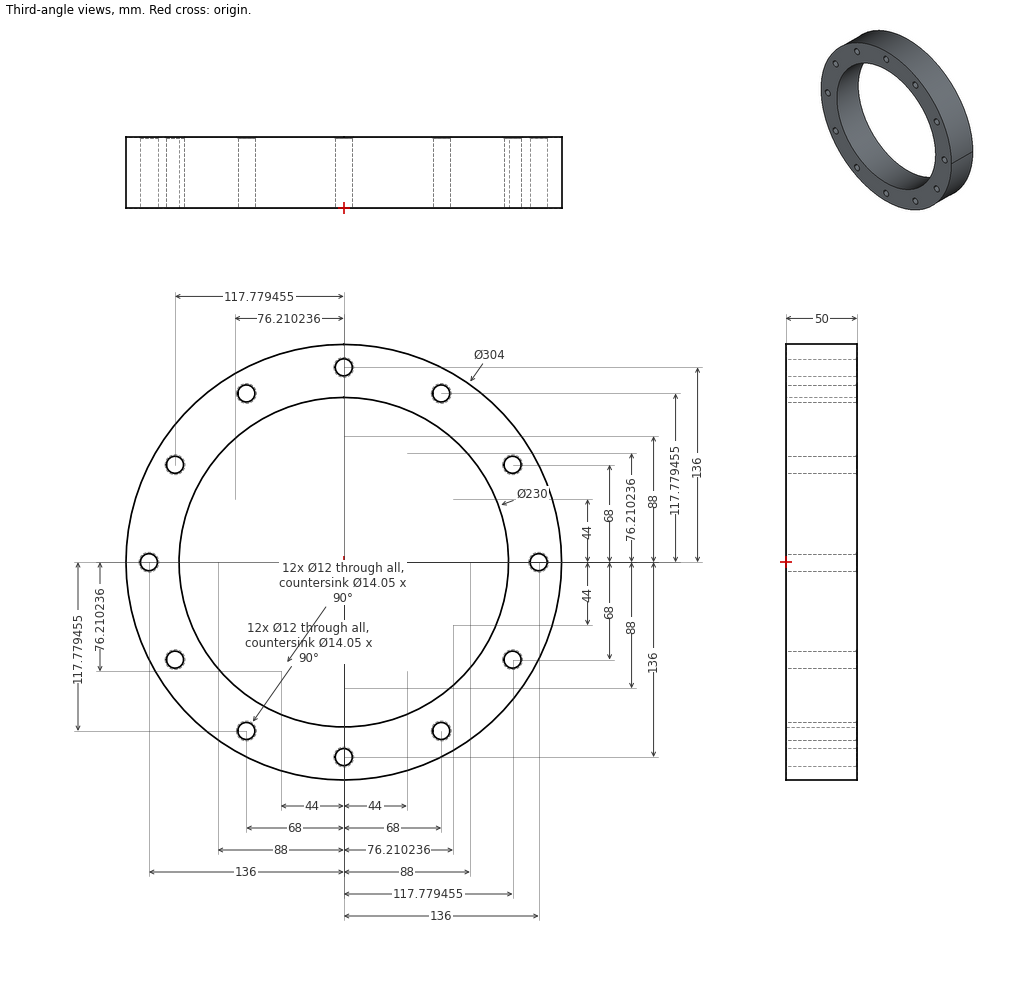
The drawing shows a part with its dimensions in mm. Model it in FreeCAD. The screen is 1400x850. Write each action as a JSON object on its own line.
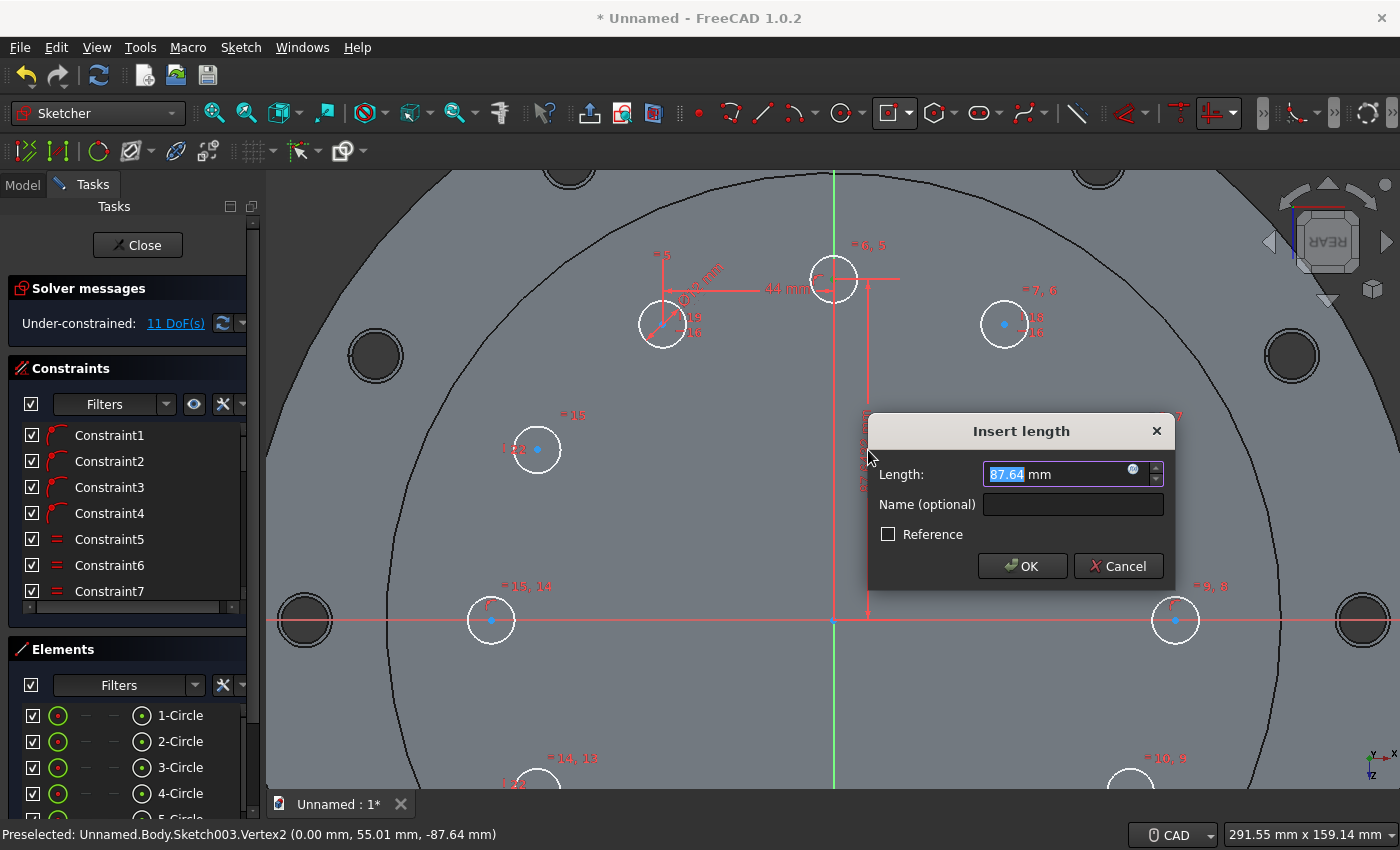
{"action": "type", "text": "88"}
{"action": "key", "text": "Return"}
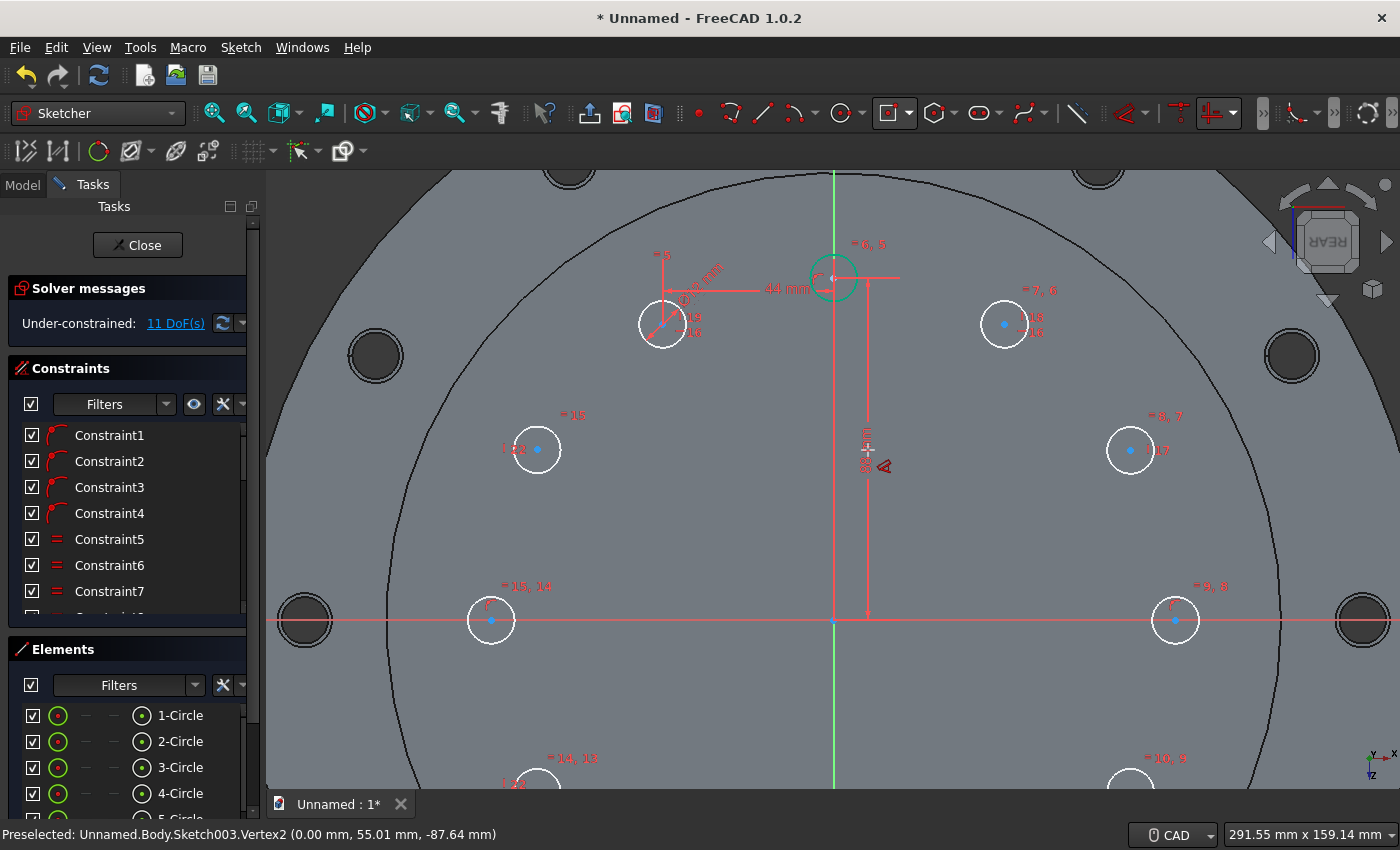
{"action": "left_click", "coordinate": [1005, 324]}
{"action": "left_click", "coordinate": [919, 290]}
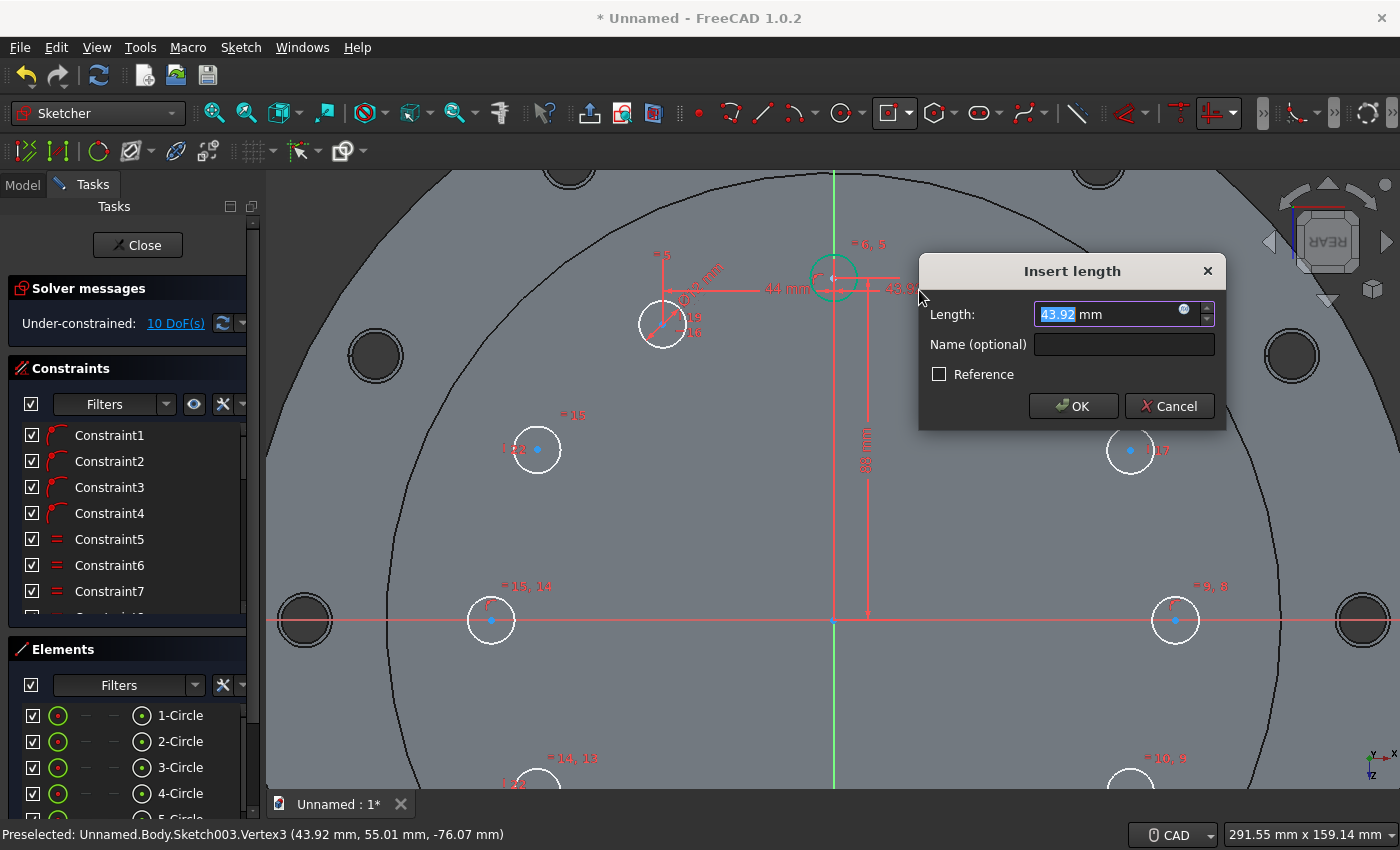
{"action": "type", "text": "44"}
{"action": "key", "text": "Return"}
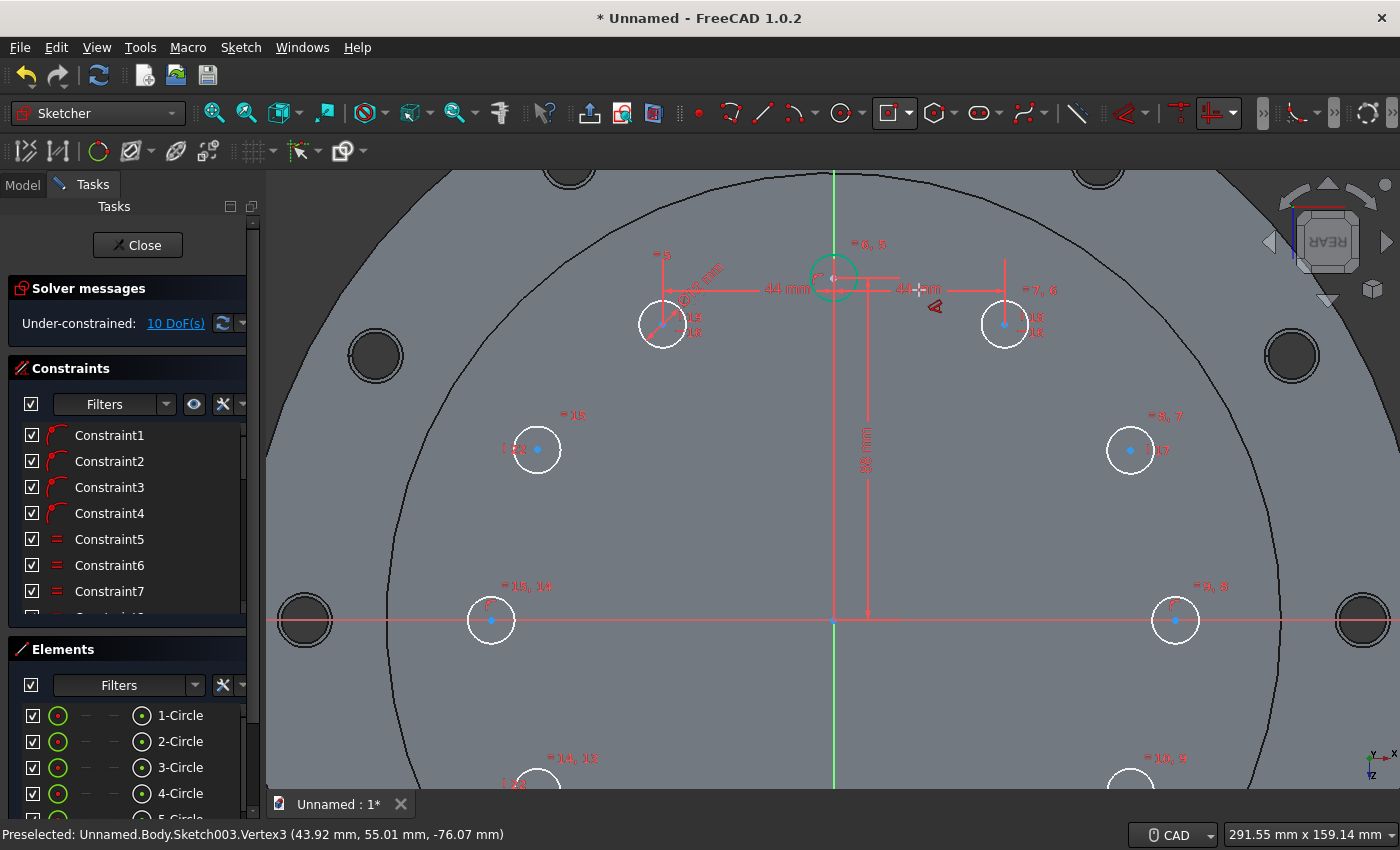
{"action": "left_click", "coordinate": [1131, 450]}
{"action": "left_click", "coordinate": [1165, 535]}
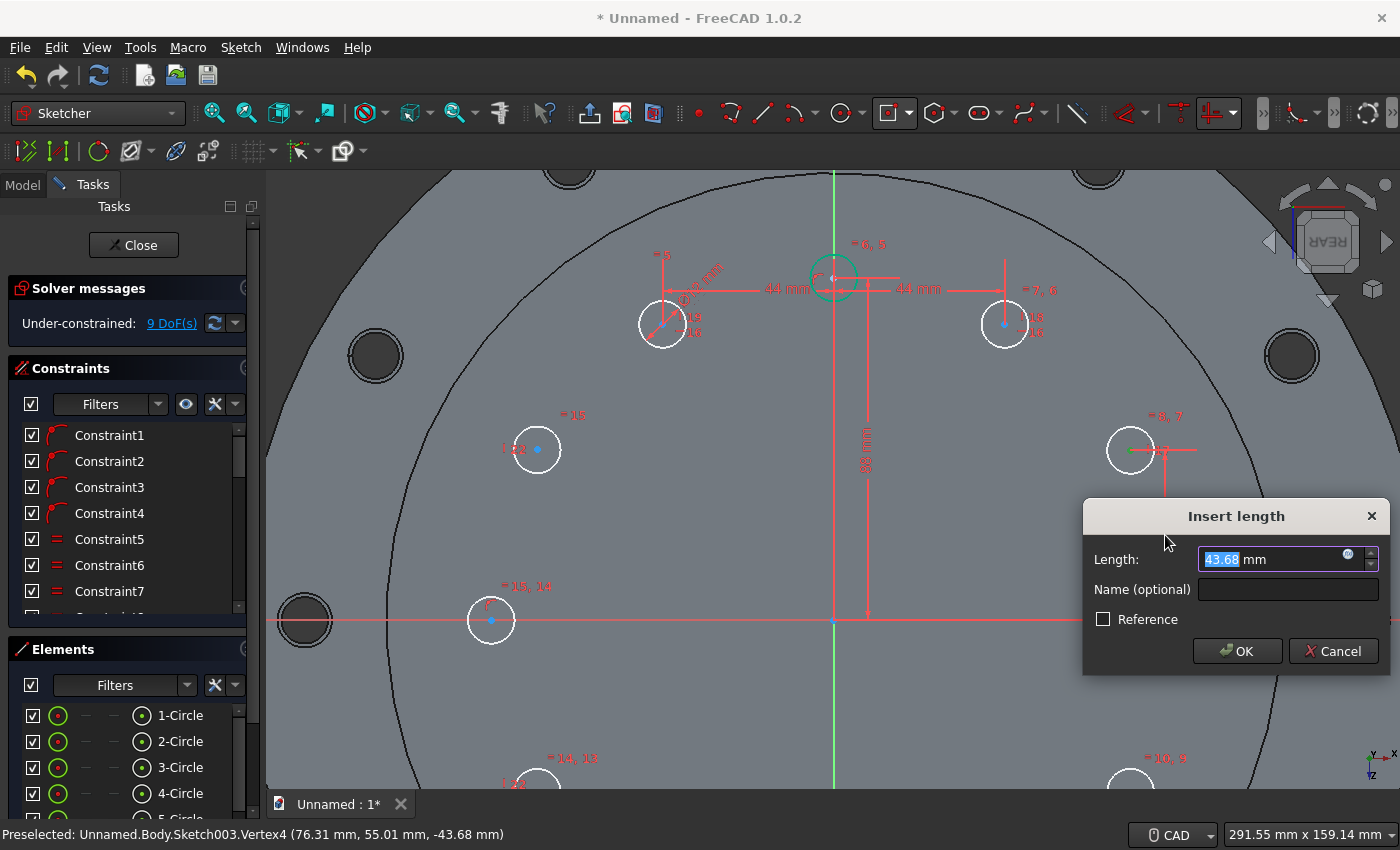
{"action": "type", "text": "44"}
{"action": "key", "text": "Return"}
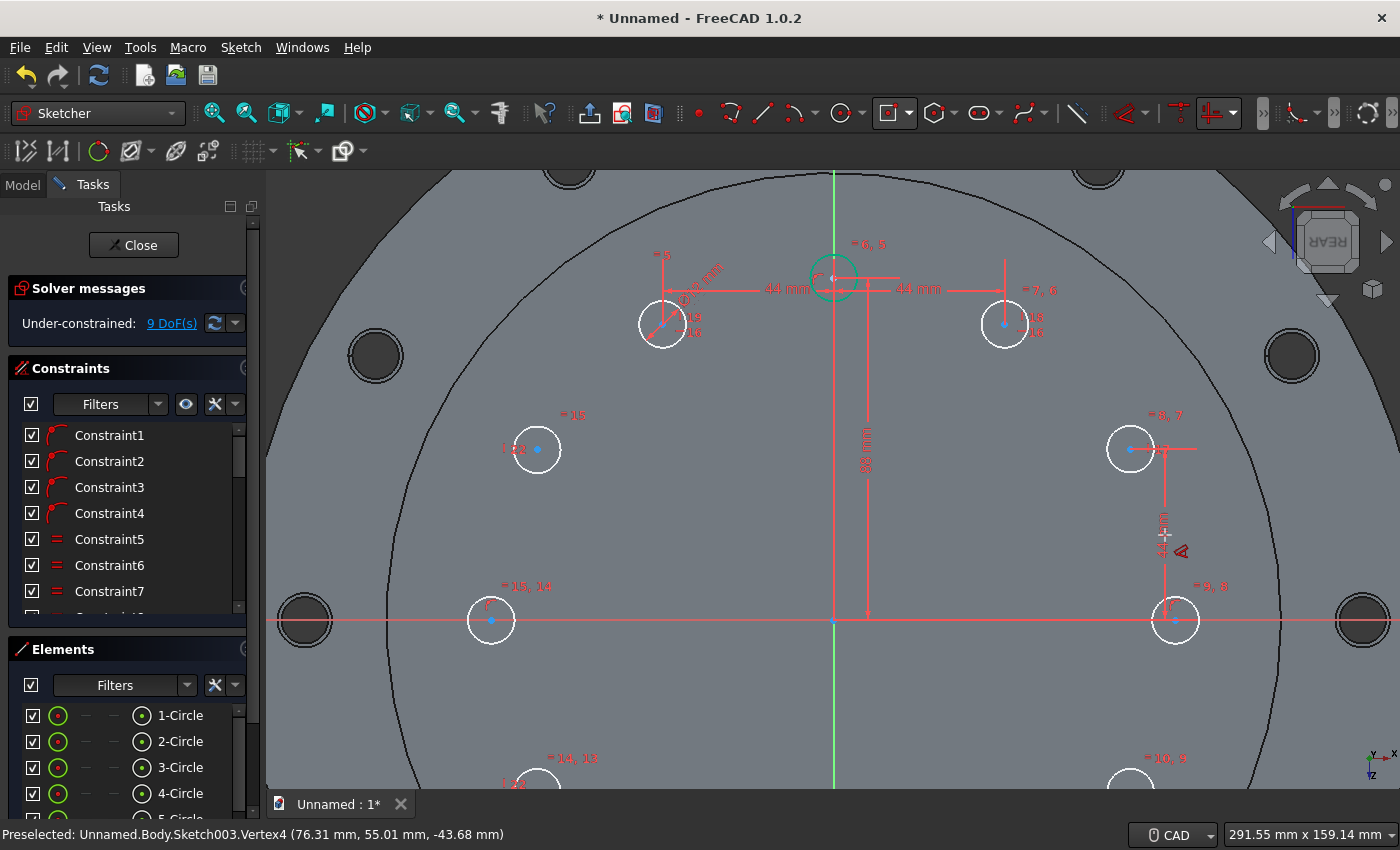
{"action": "left_click", "coordinate": [1176, 620]}
{"action": "left_click", "coordinate": [1005, 654]}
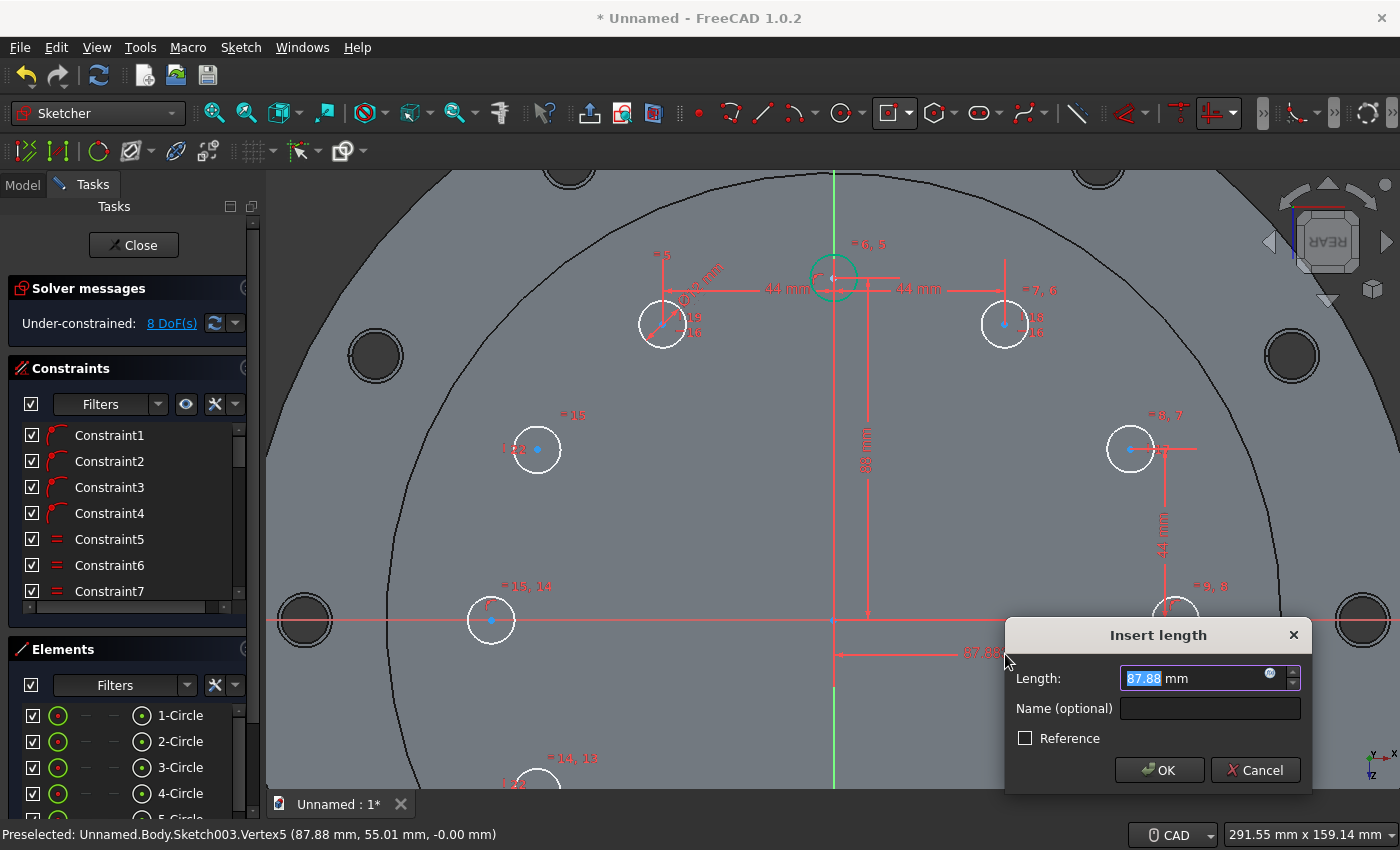
{"action": "type", "text": "88"}
{"action": "key", "text": "Return"}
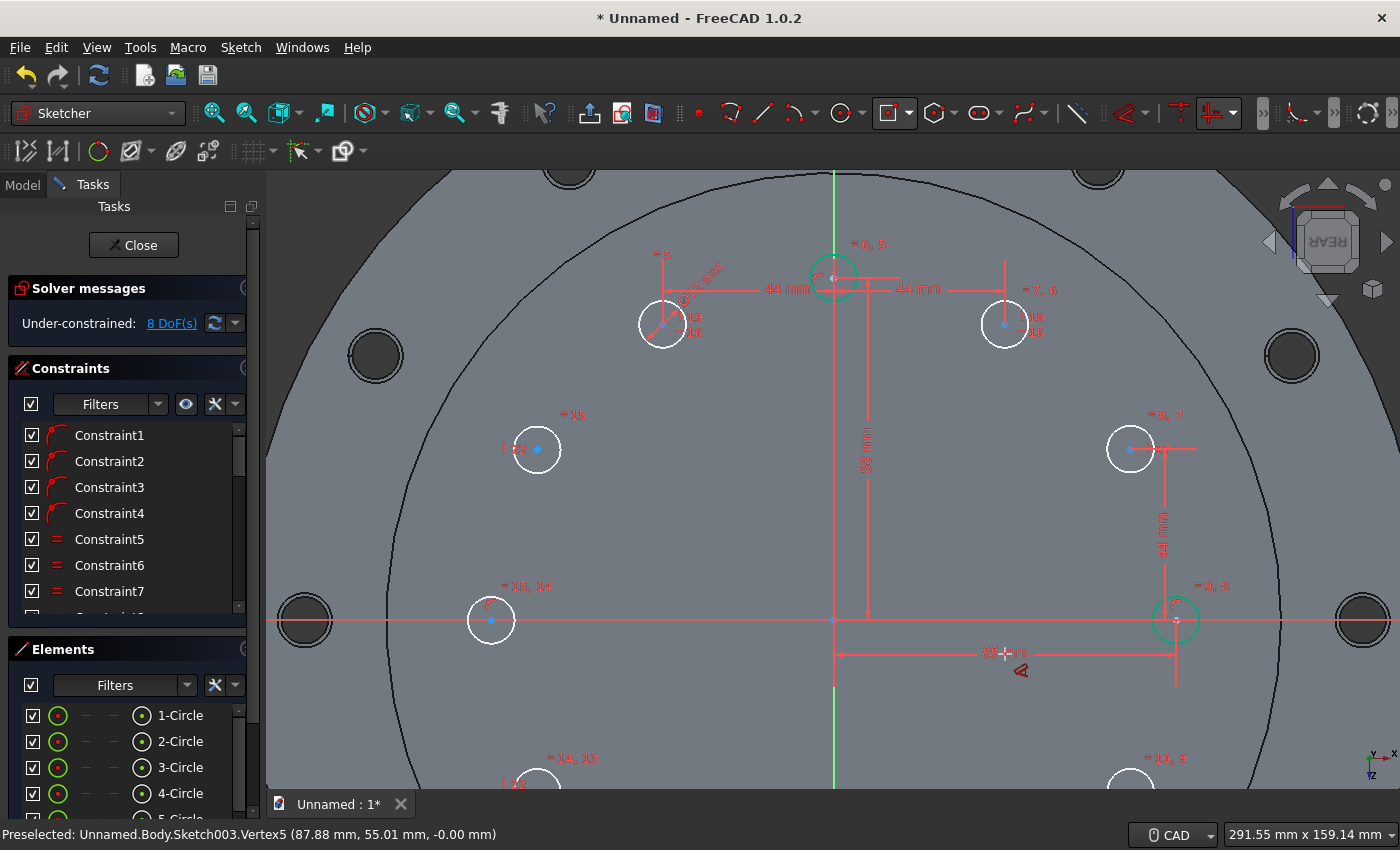
{"action": "scroll", "coordinate": [680, 308], "scroll_direction": "down", "scroll_amount": 3}